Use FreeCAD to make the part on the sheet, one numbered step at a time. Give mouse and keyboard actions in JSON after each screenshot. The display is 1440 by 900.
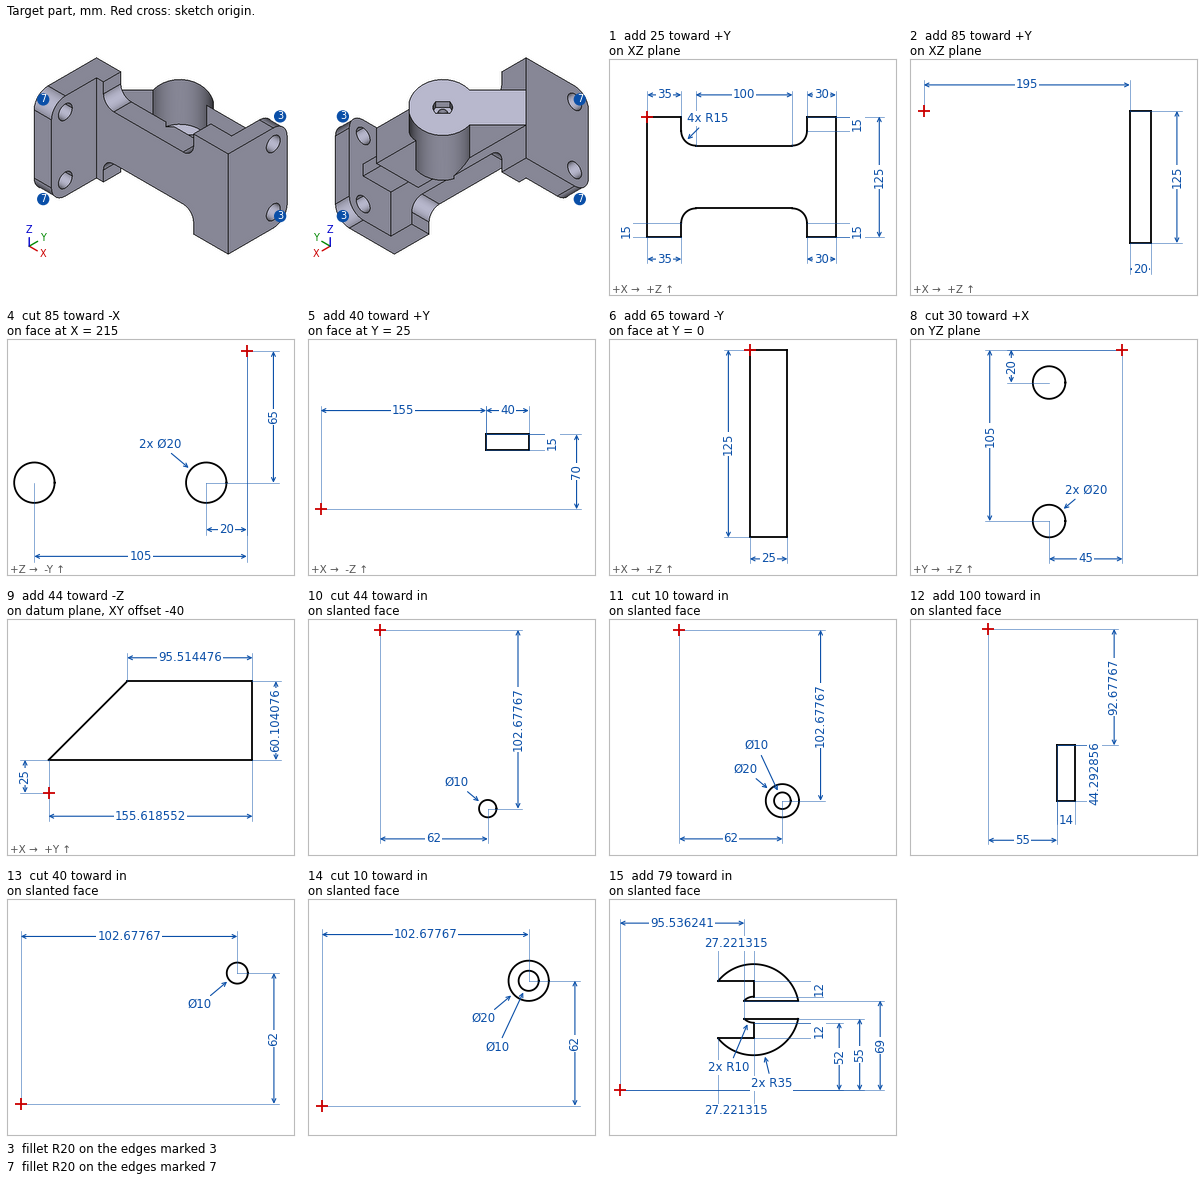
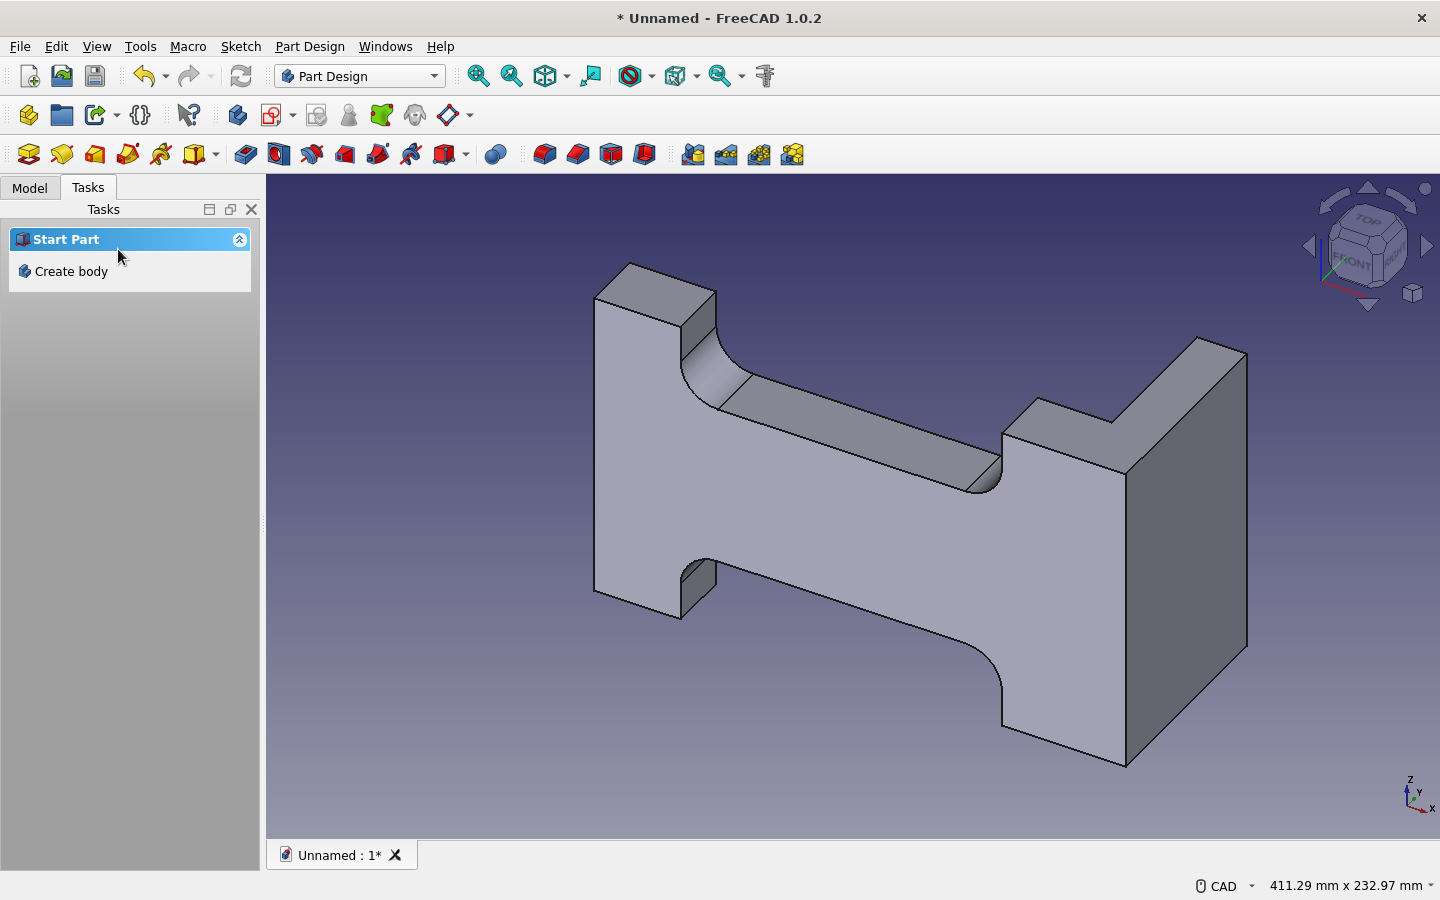
{"action": "key", "text": "0"}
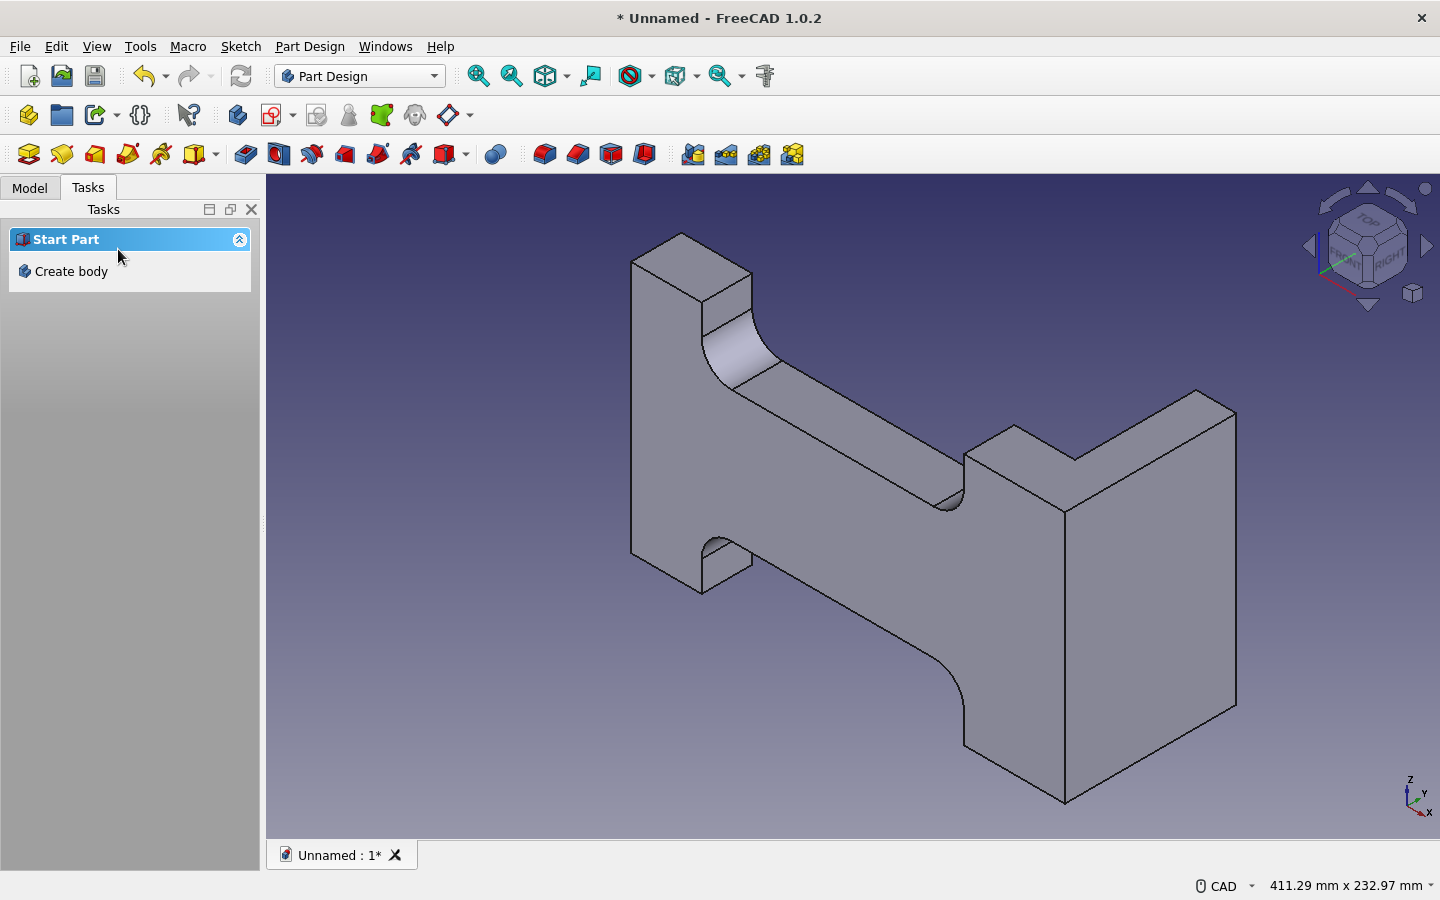
{"action": "left_click", "coordinate": [479, 76]}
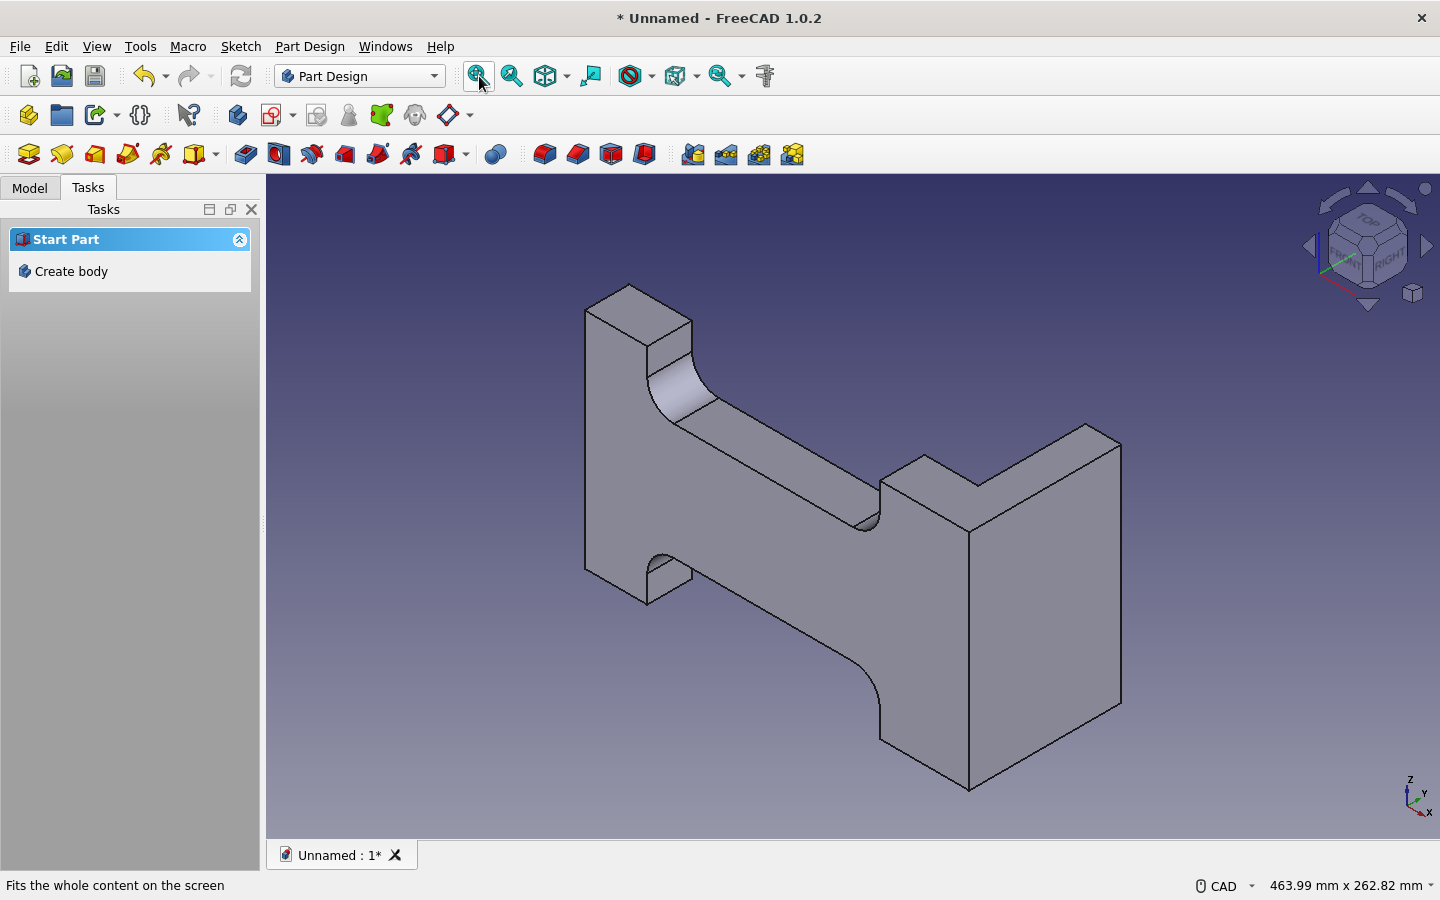
{"action": "key", "text": "2"}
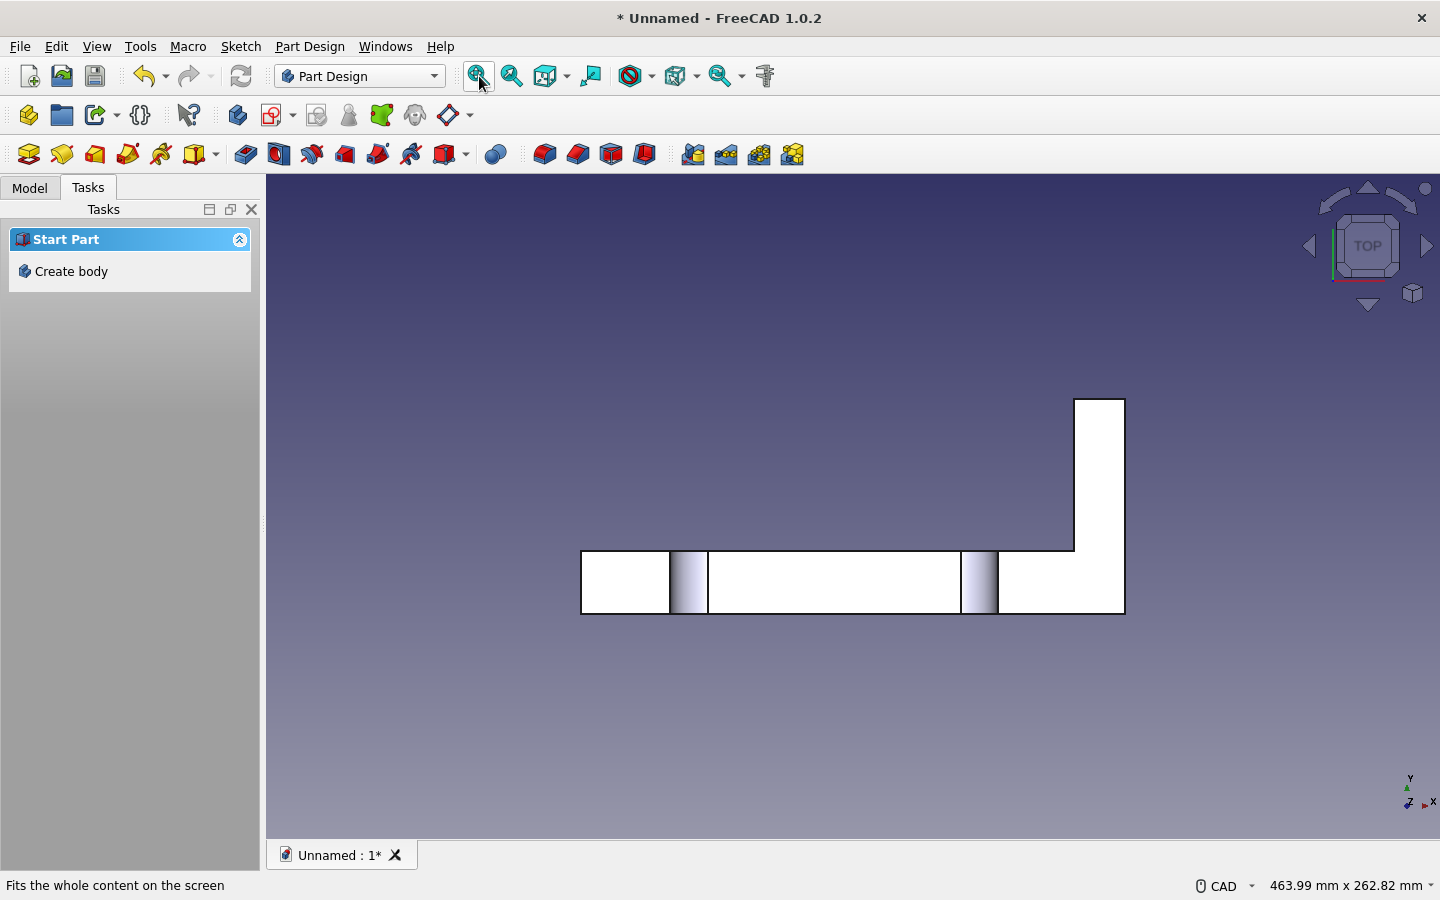
{"action": "left_click", "coordinate": [1100, 398]}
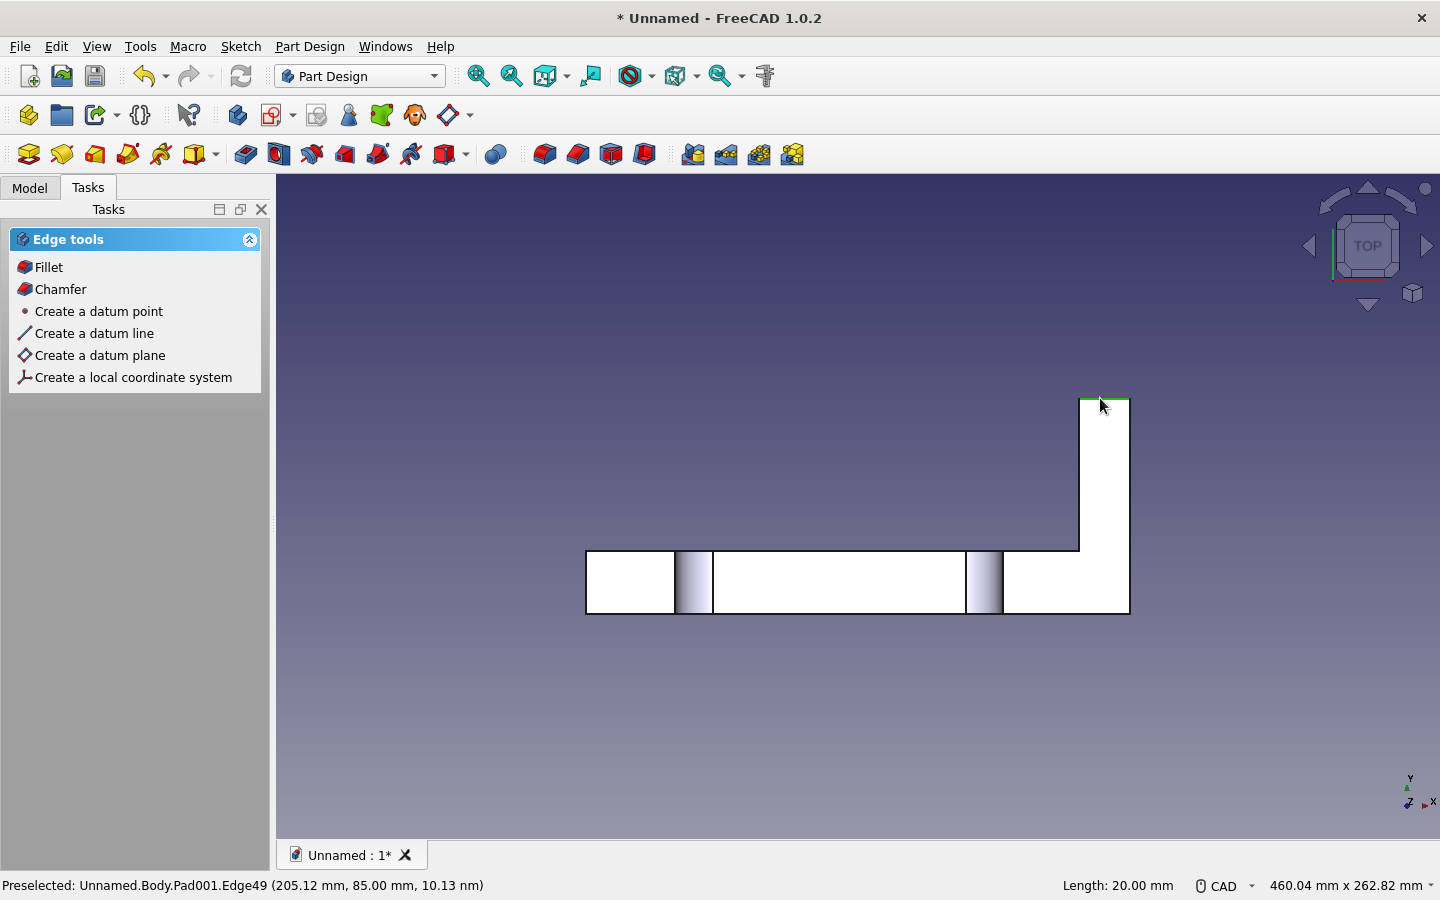
{"action": "key", "text": "1"}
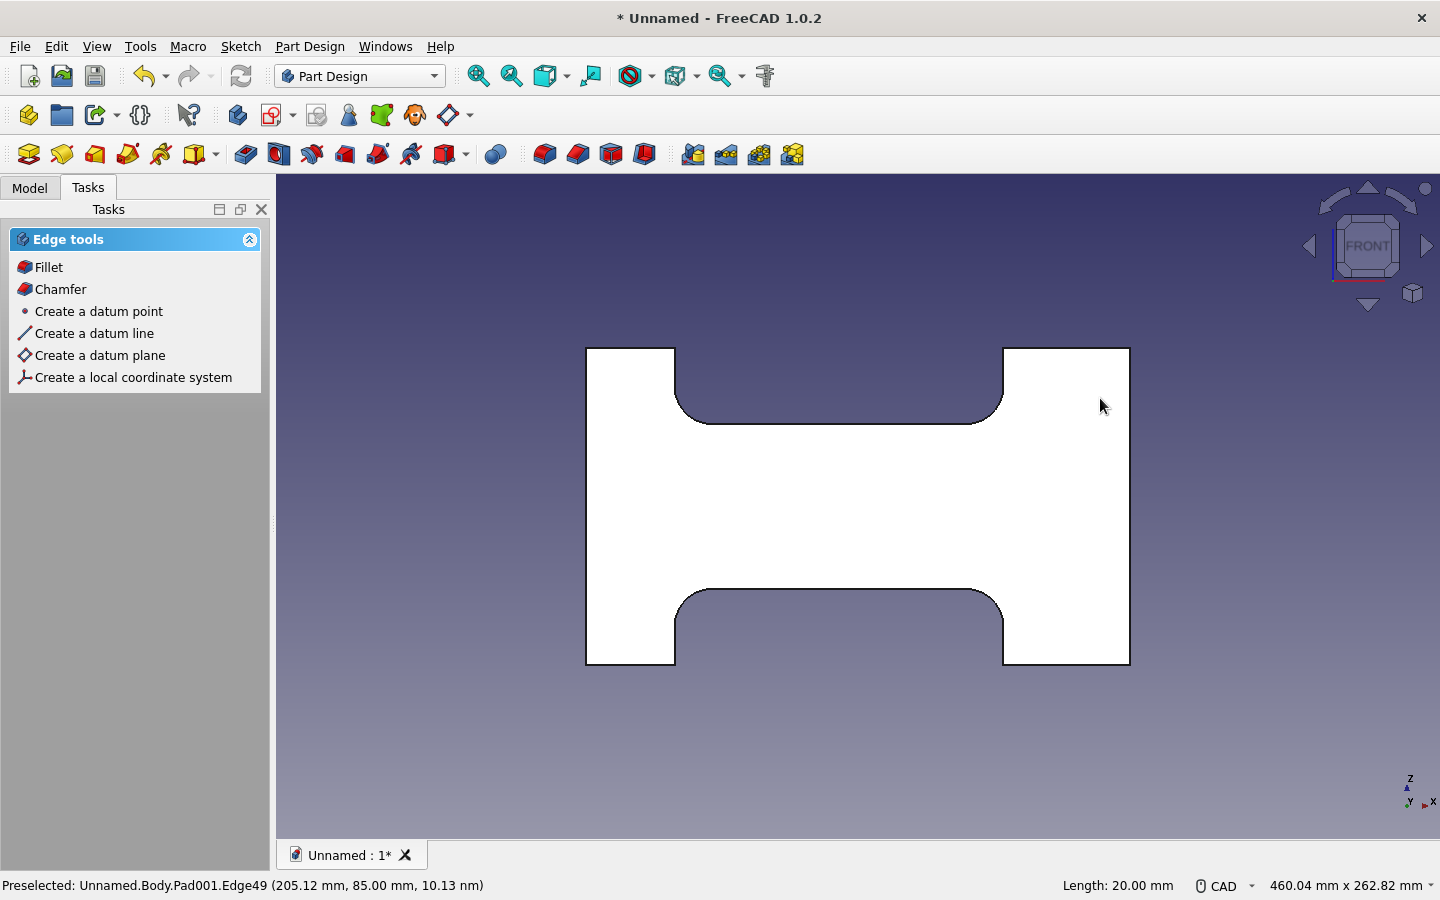
{"action": "key", "text": "3"}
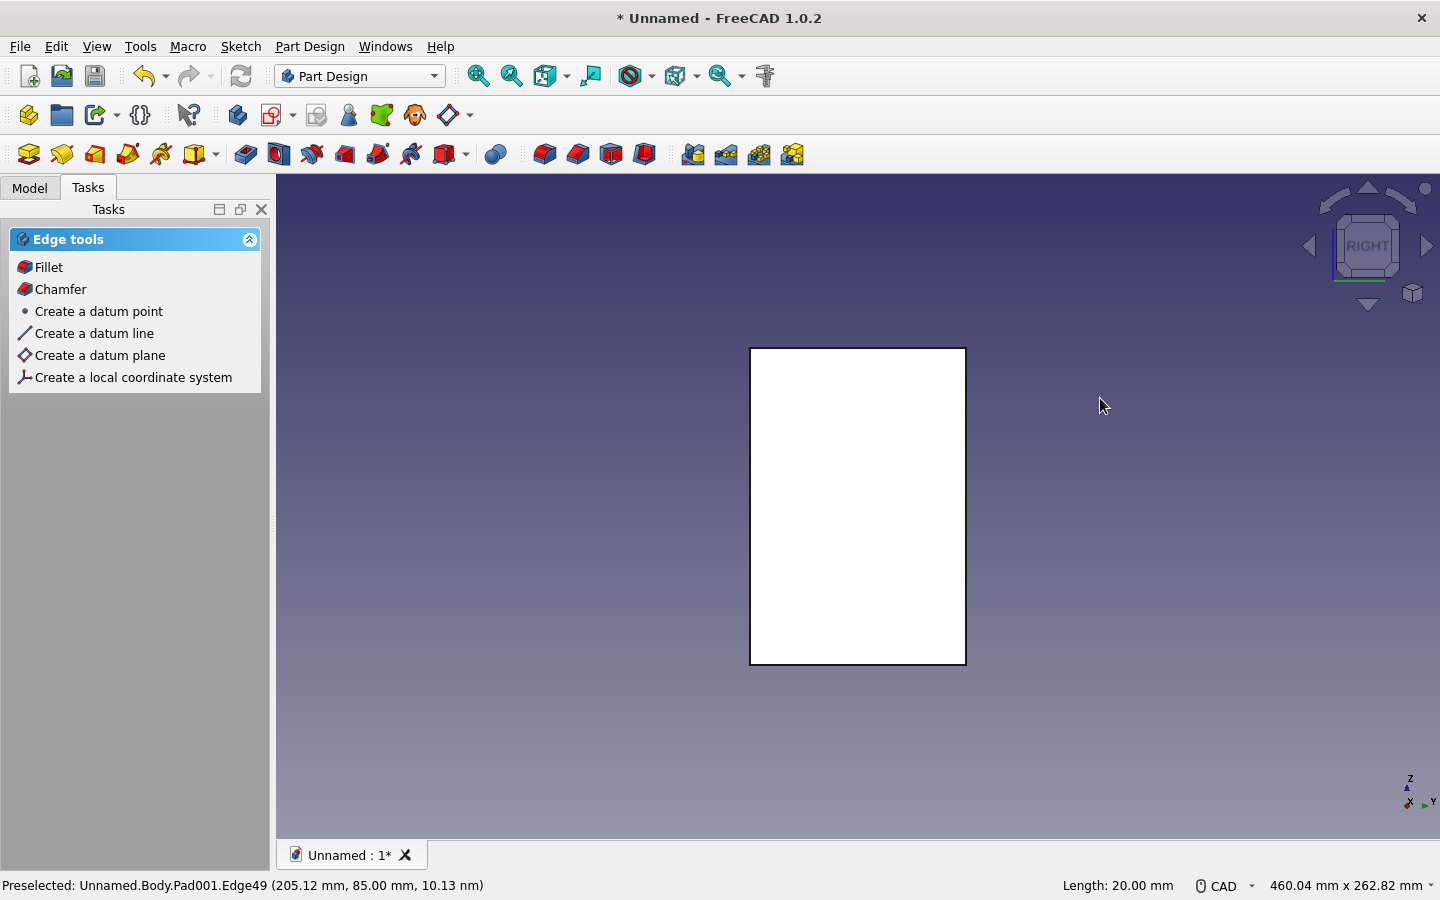
{"action": "key", "text": "5"}